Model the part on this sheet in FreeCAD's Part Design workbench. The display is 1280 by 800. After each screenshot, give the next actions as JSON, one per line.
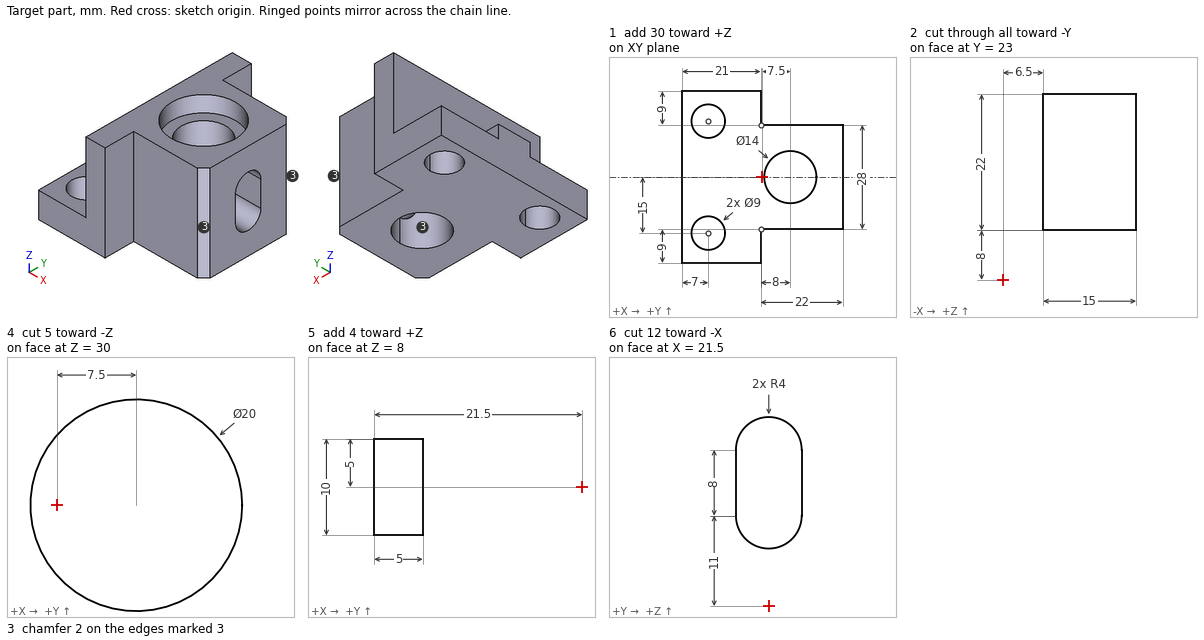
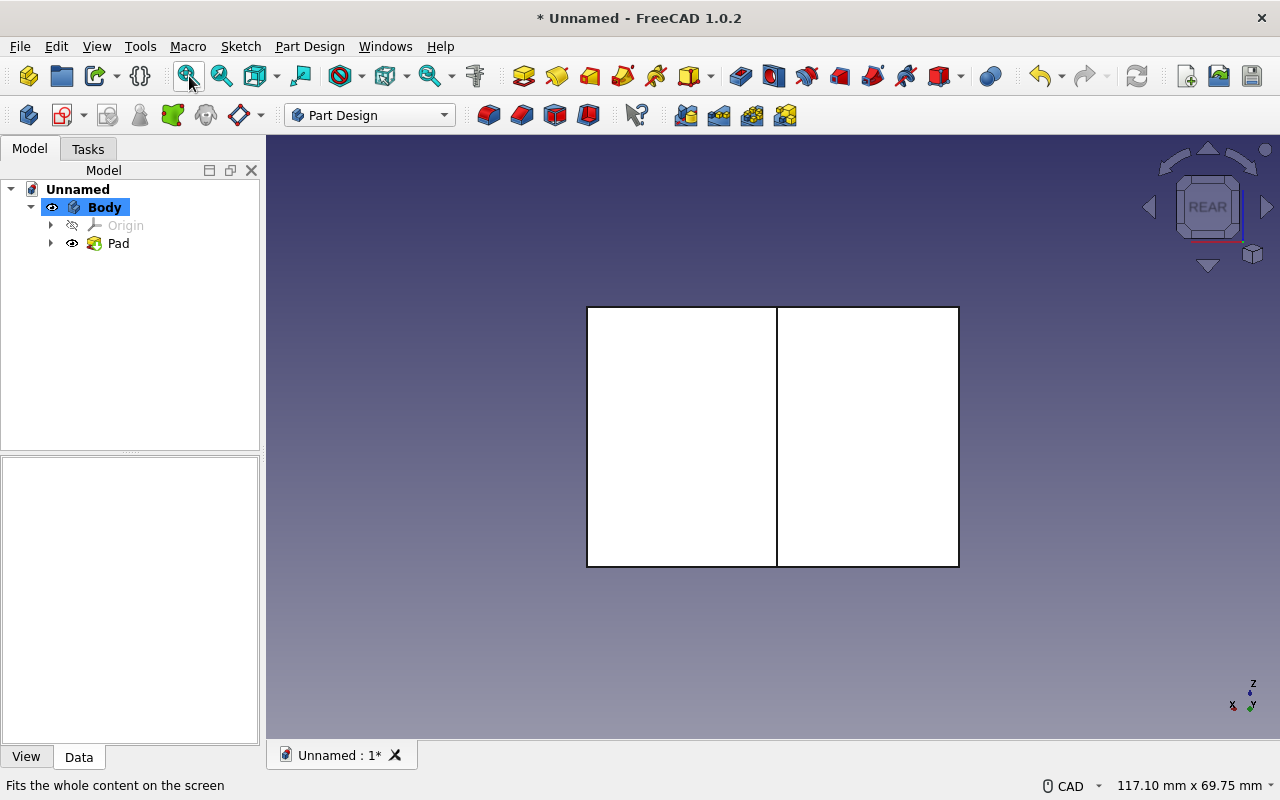
{"action": "left_click", "coordinate": [868, 399]}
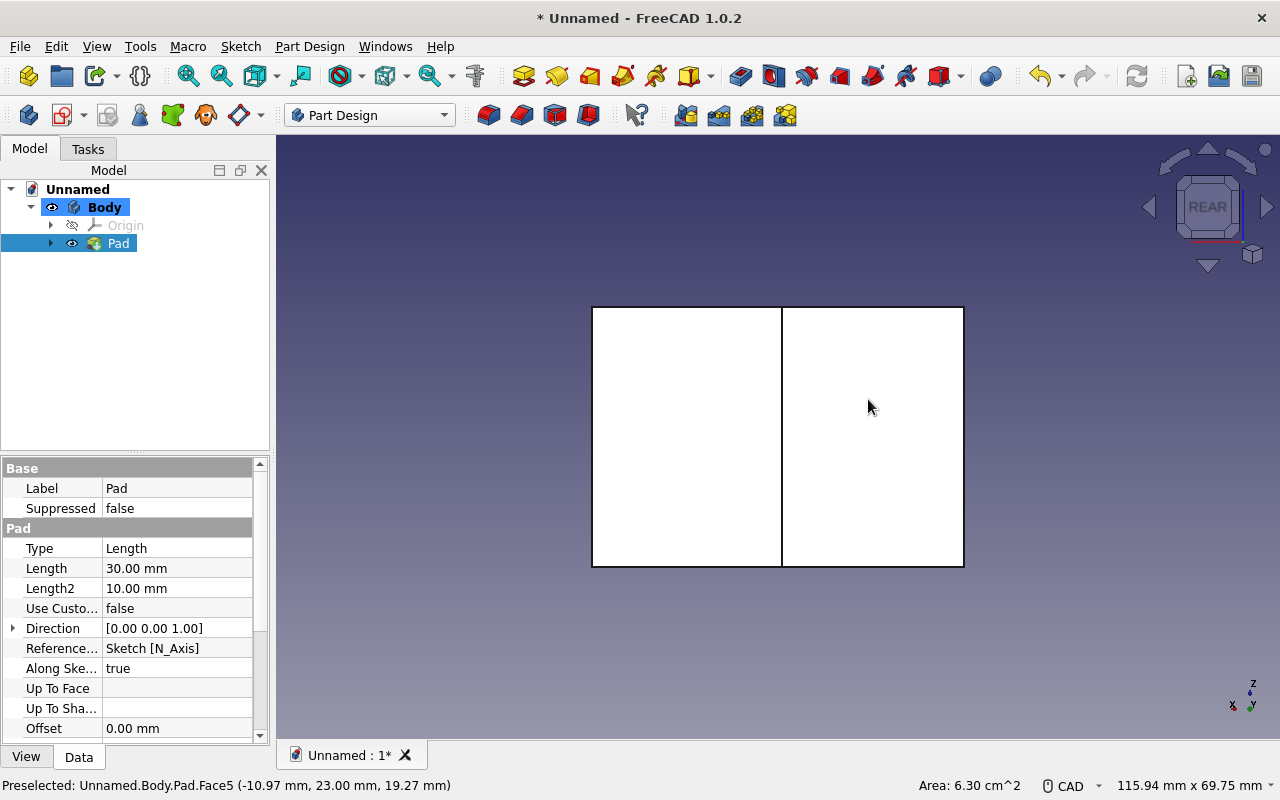
{"action": "left_click", "coordinate": [62, 116]}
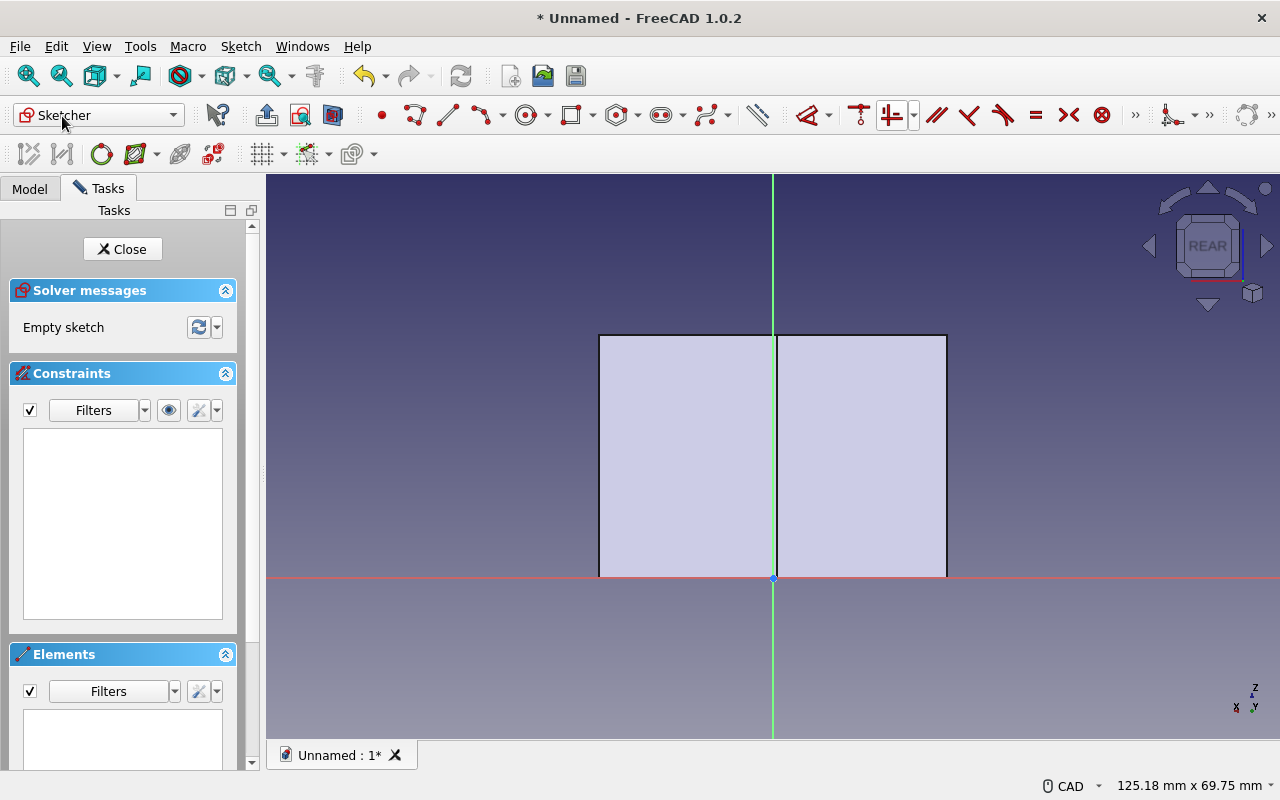
{"action": "scroll", "coordinate": [1115, 457], "scroll_direction": "up", "scroll_amount": 2}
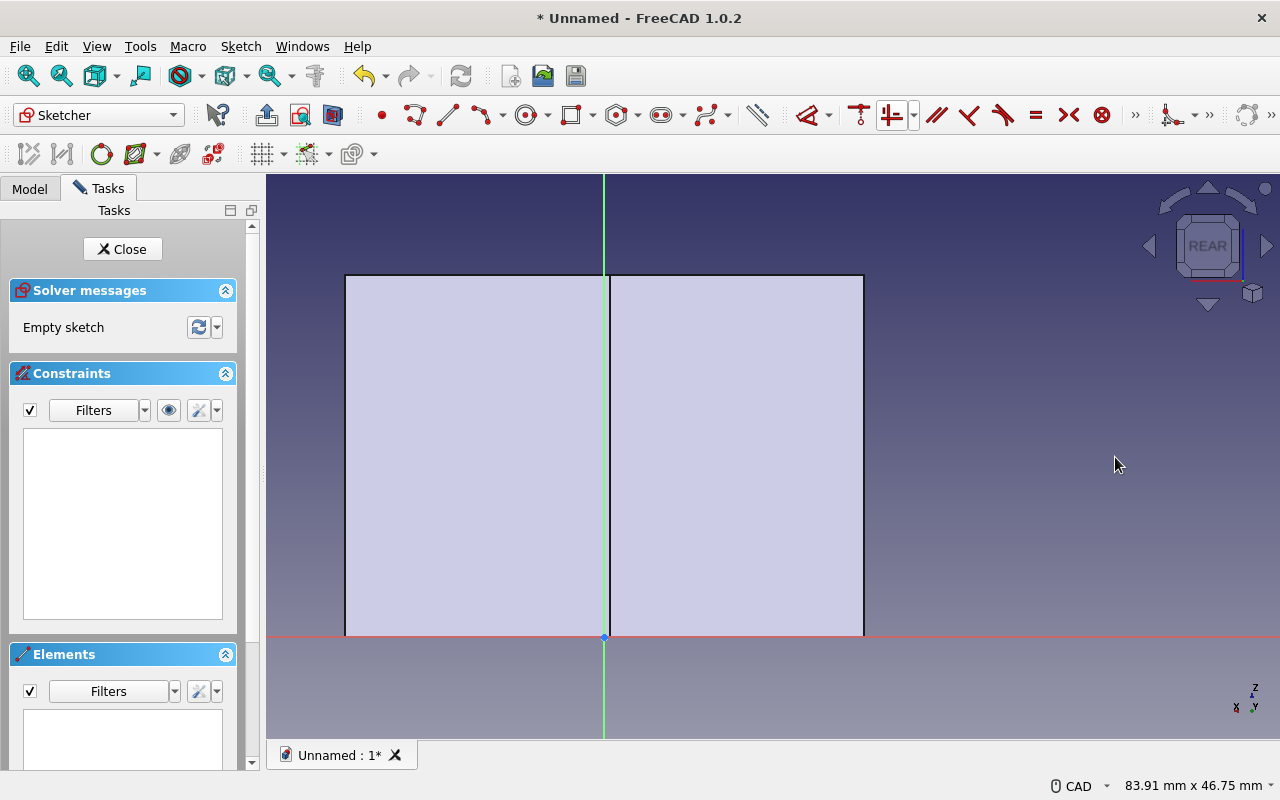
{"action": "key", "text": "g r"}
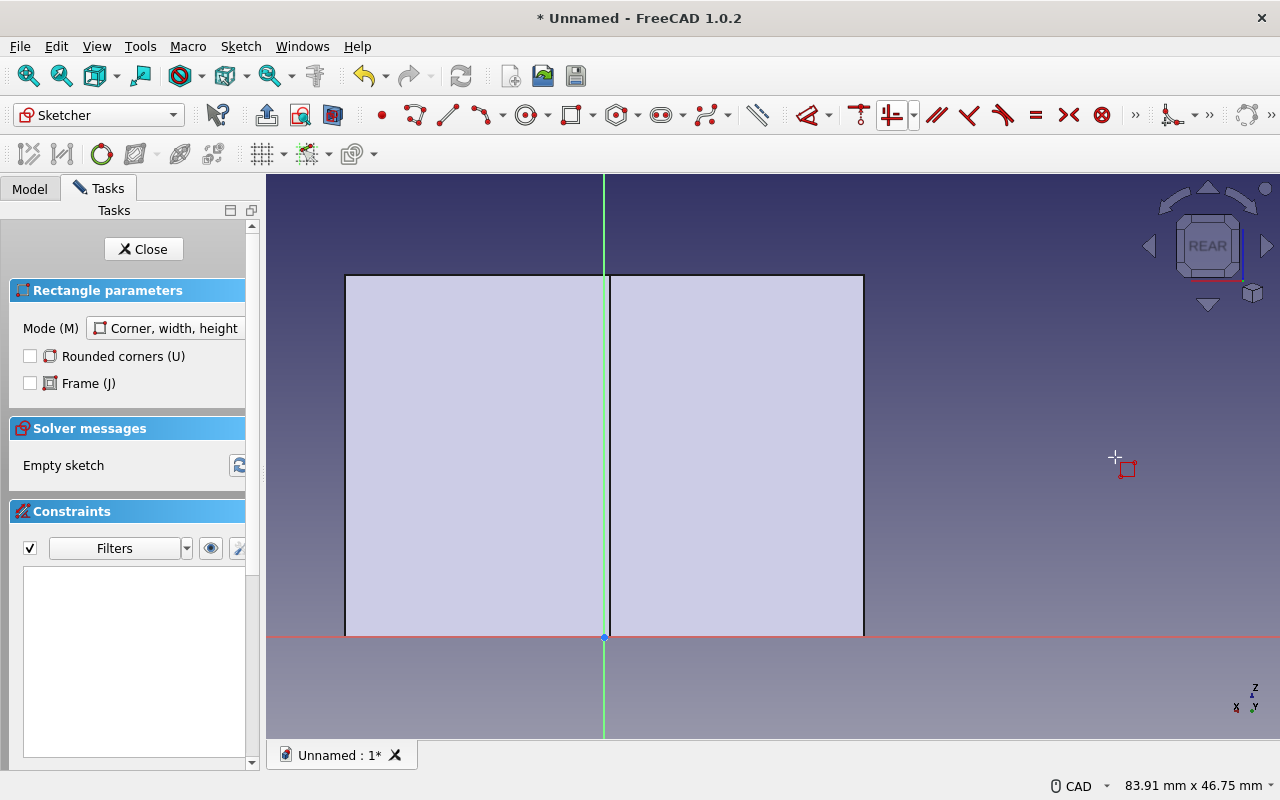
{"action": "left_click", "coordinate": [683, 275]}
{"action": "left_click", "coordinate": [864, 541]}
{"action": "key", "text": "Escape"}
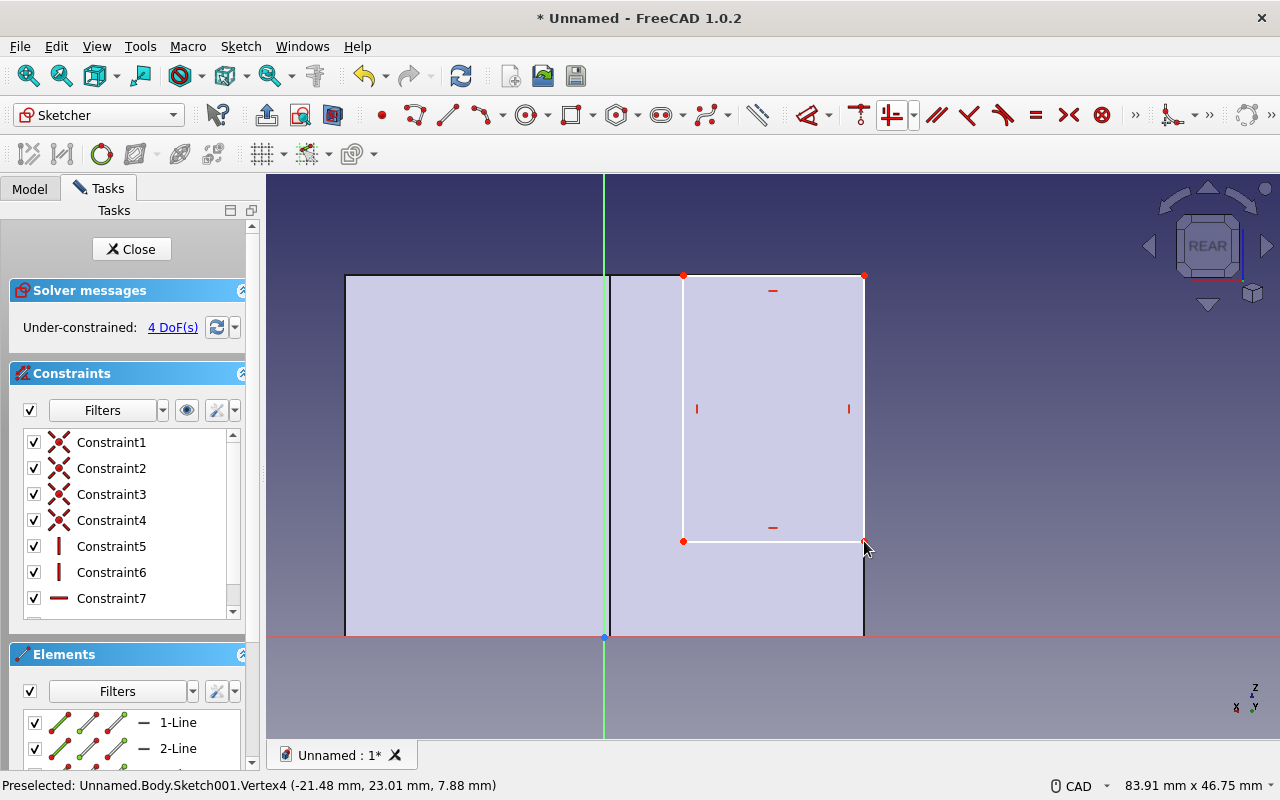
{"action": "key", "text": "d"}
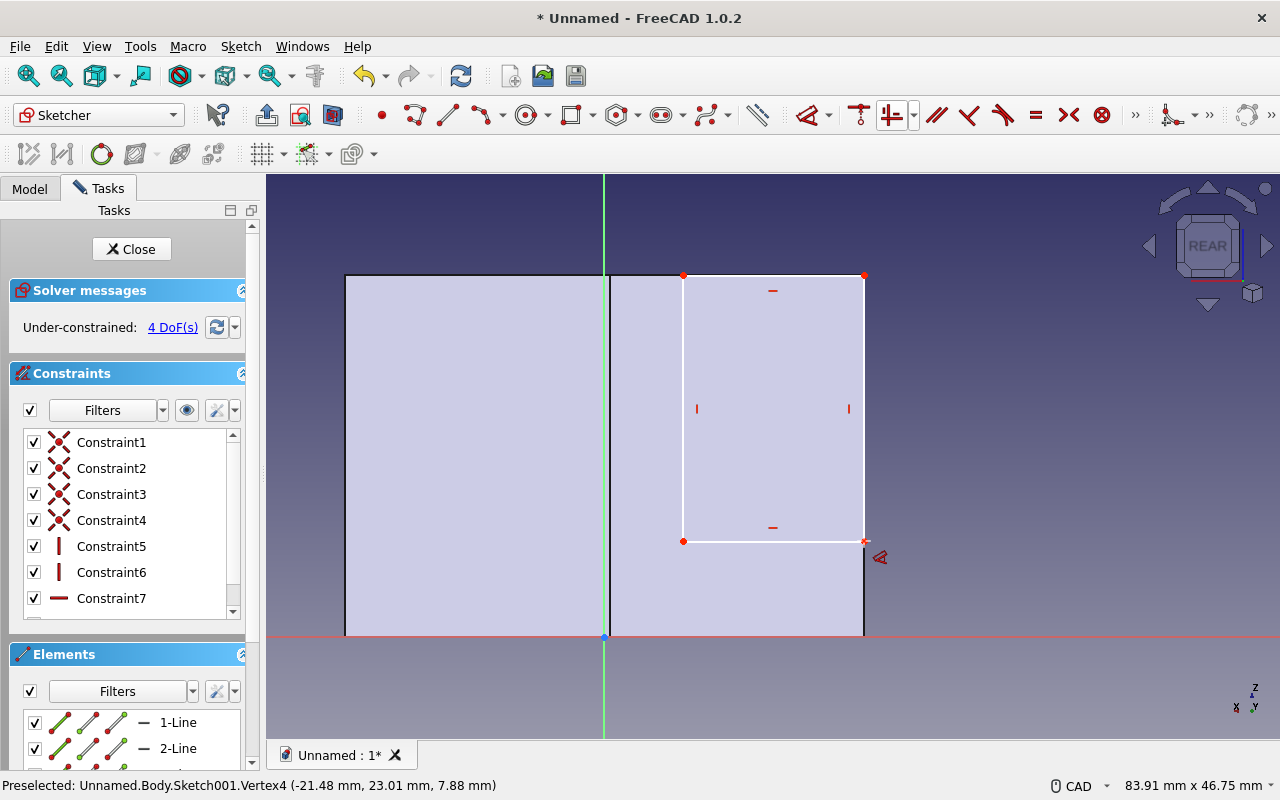
{"action": "left_click", "coordinate": [683, 356]}
{"action": "left_click", "coordinate": [649, 409]}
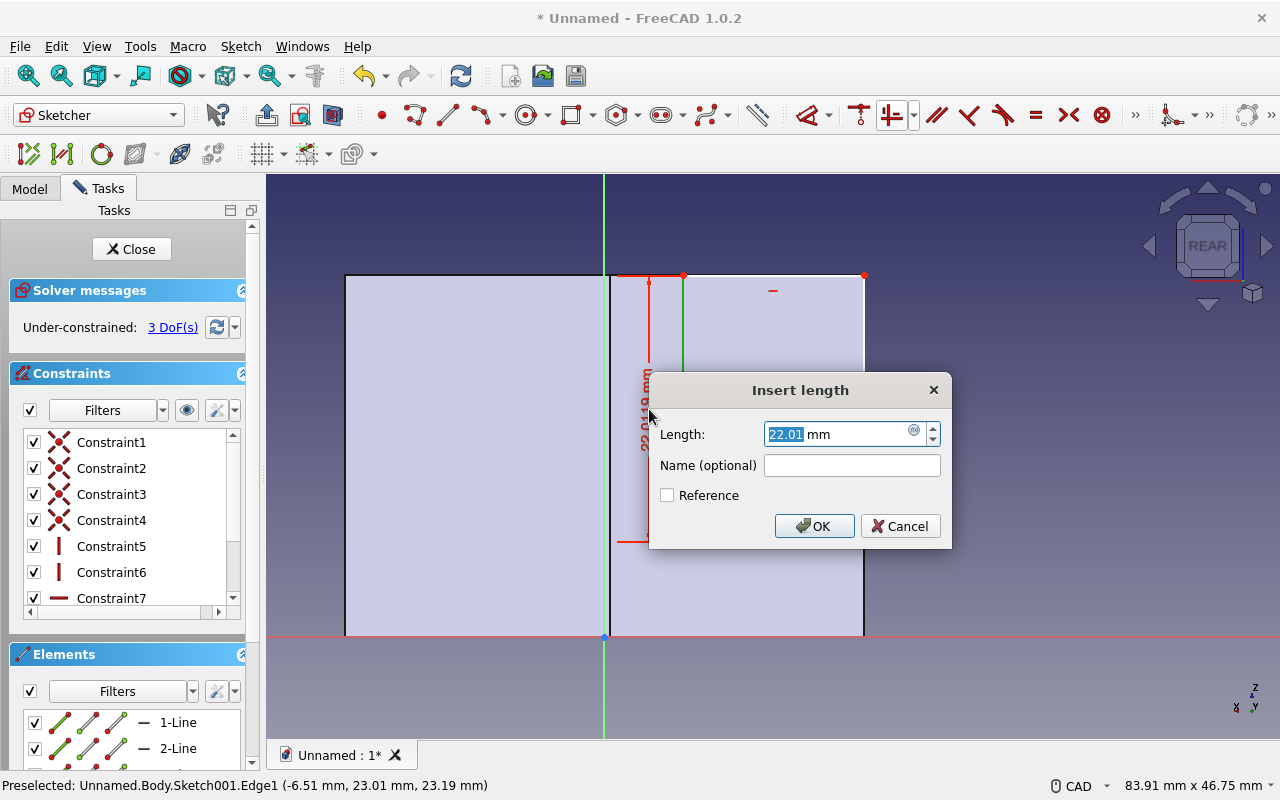
{"action": "type", "text": "22"}
{"action": "key", "text": "Return"}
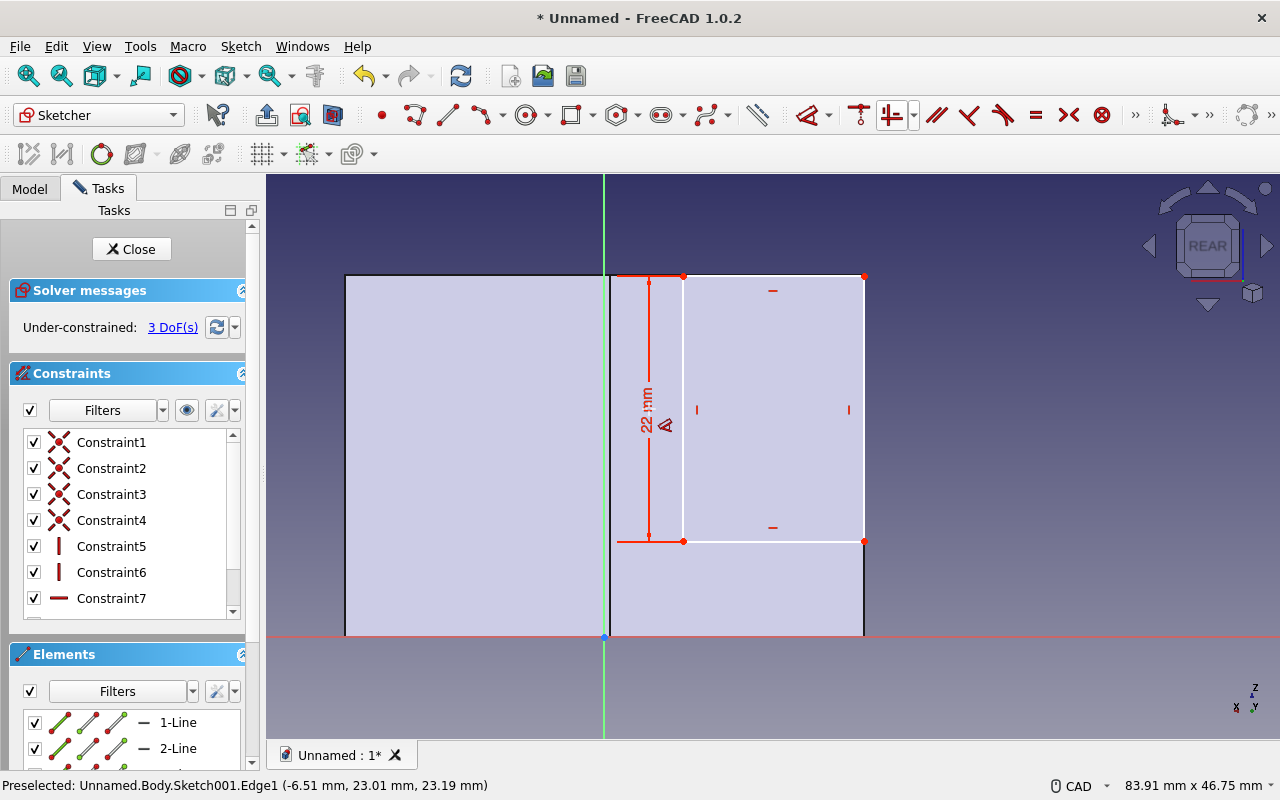
{"action": "left_click", "coordinate": [737, 542]}
{"action": "left_click", "coordinate": [774, 576]}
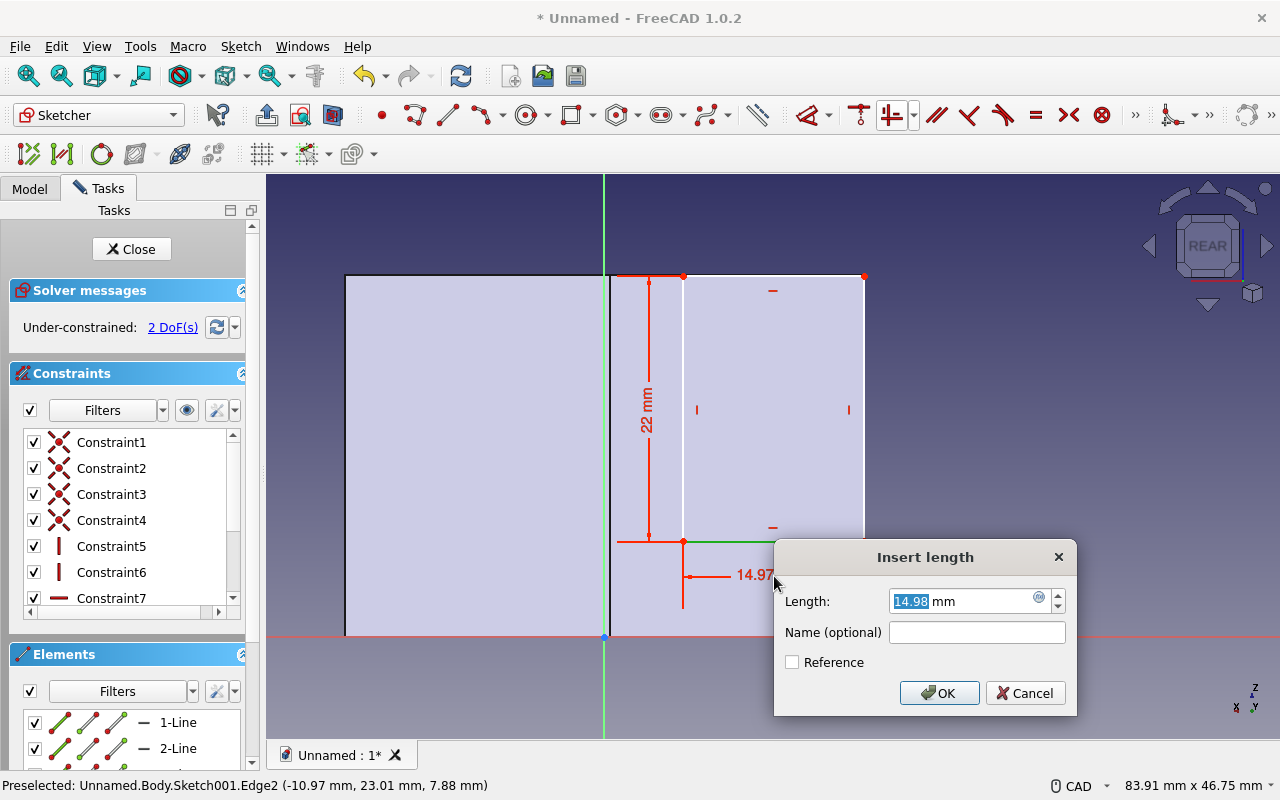
{"action": "type", "text": "15"}
{"action": "key", "text": "Return"}